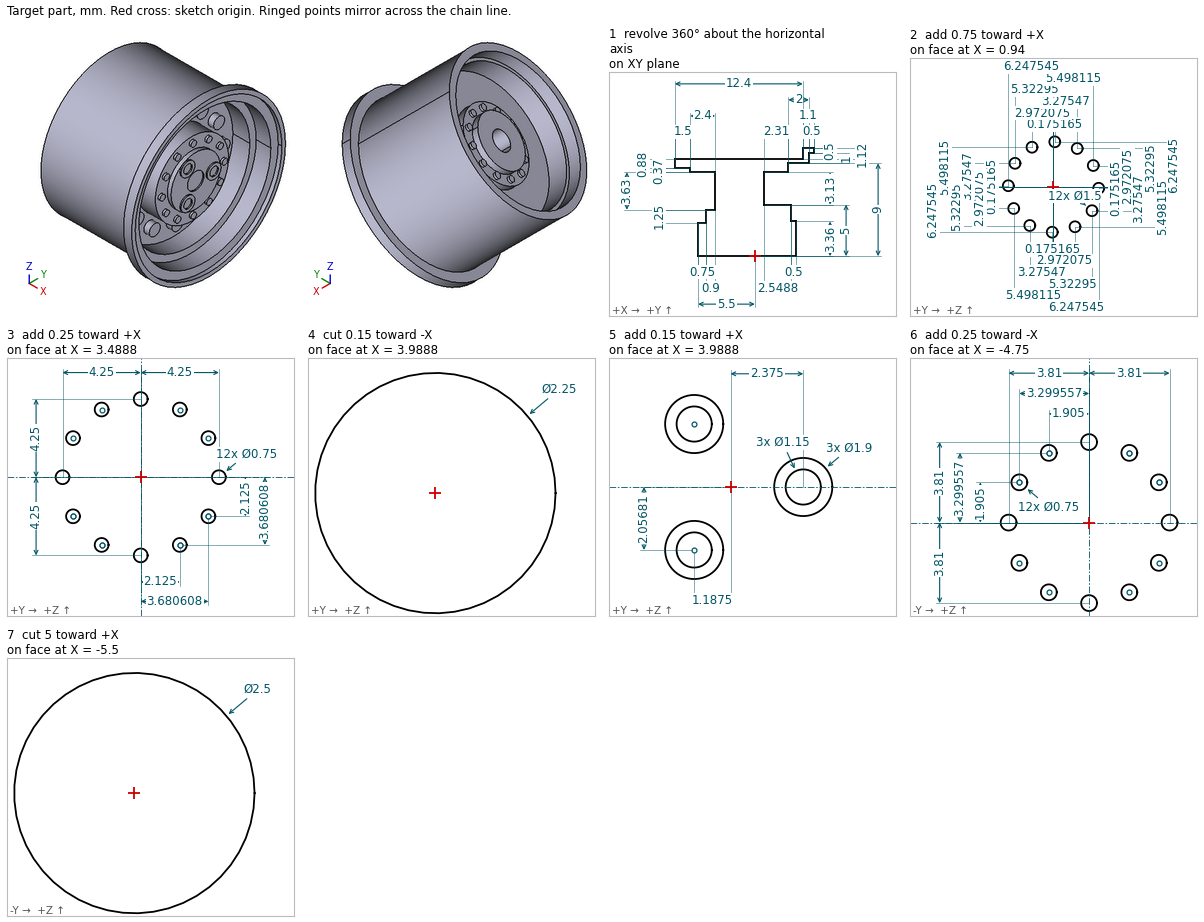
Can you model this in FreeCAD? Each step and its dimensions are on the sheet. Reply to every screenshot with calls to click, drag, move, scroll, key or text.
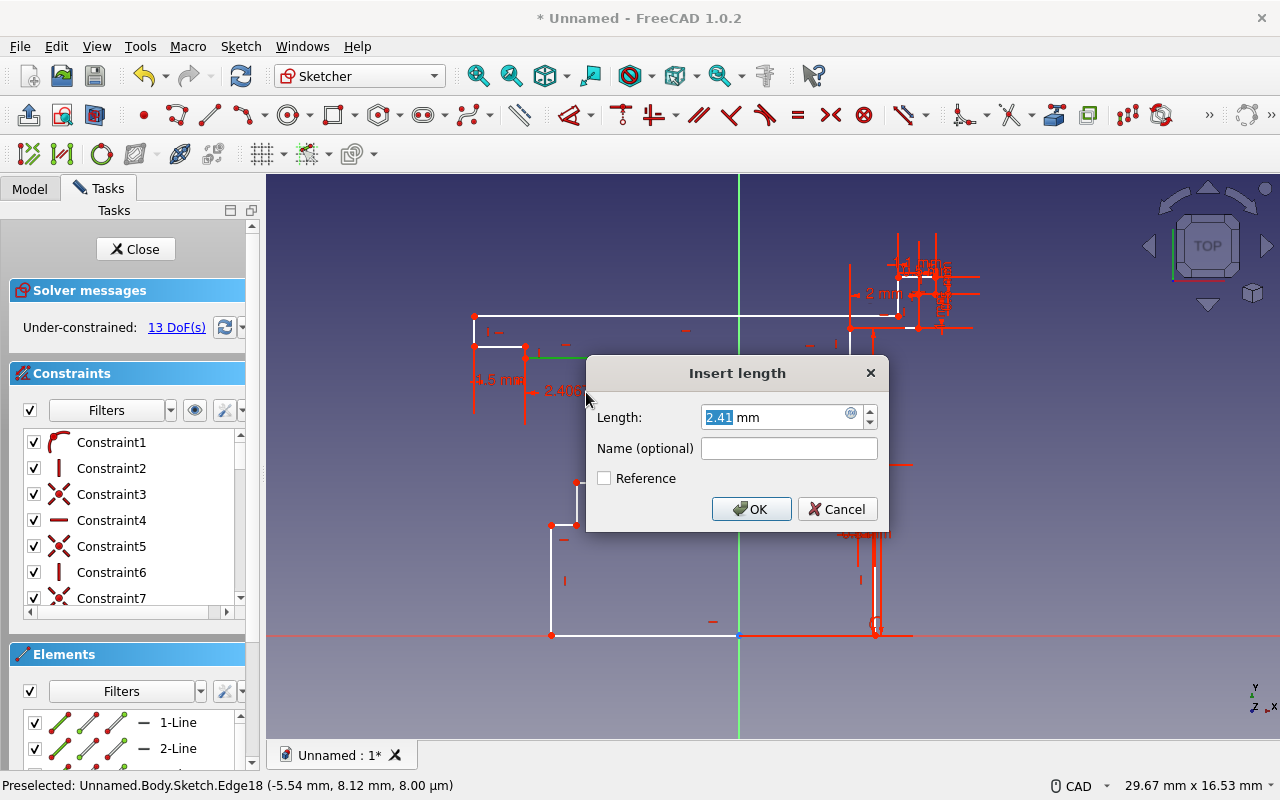
text(2.4)
key(Return)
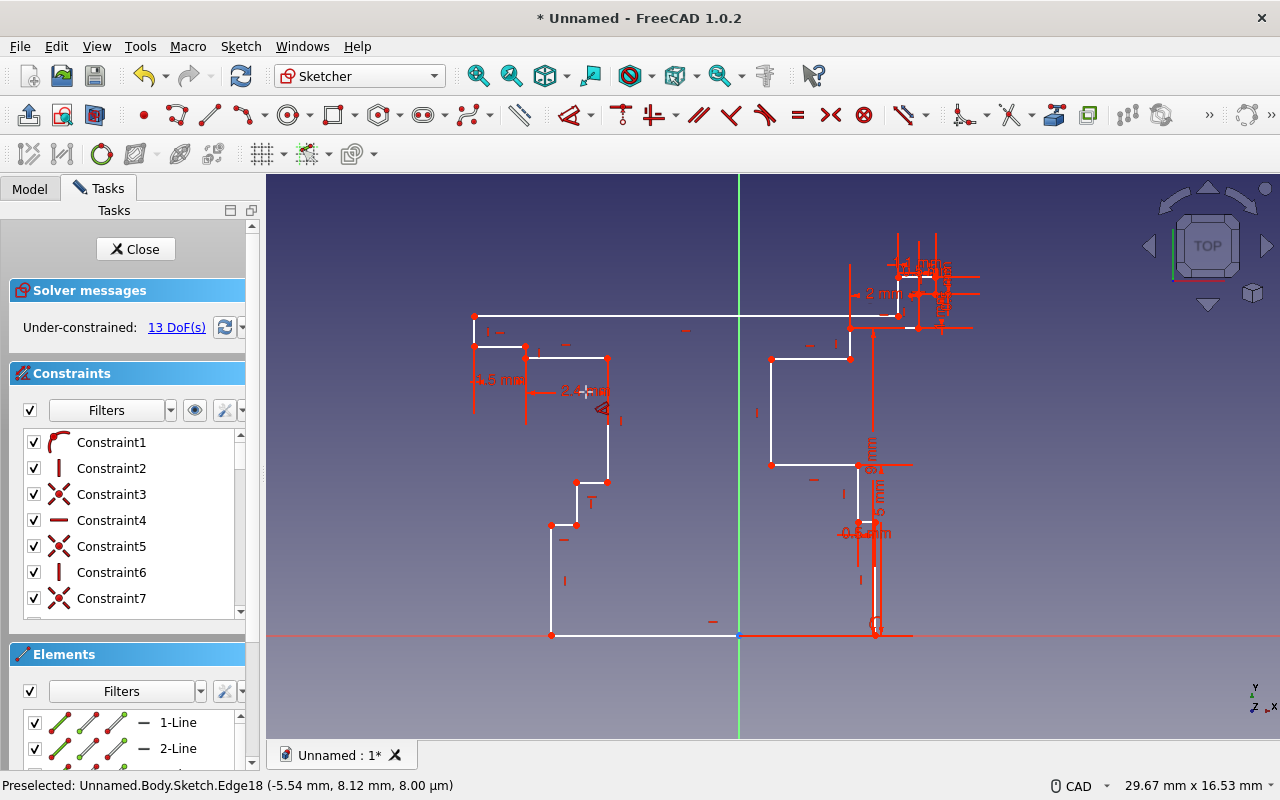
scroll(599, 483, up, 3)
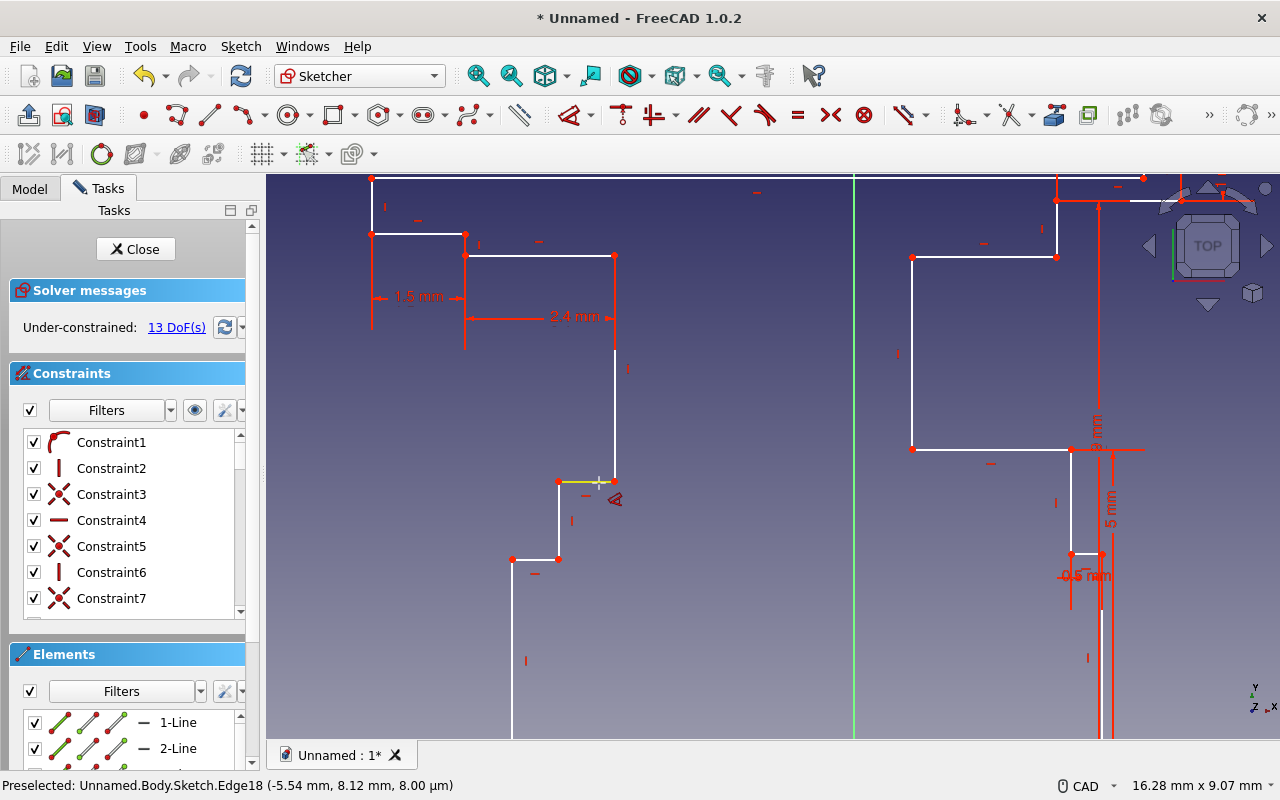
click(598, 482)
click(587, 516)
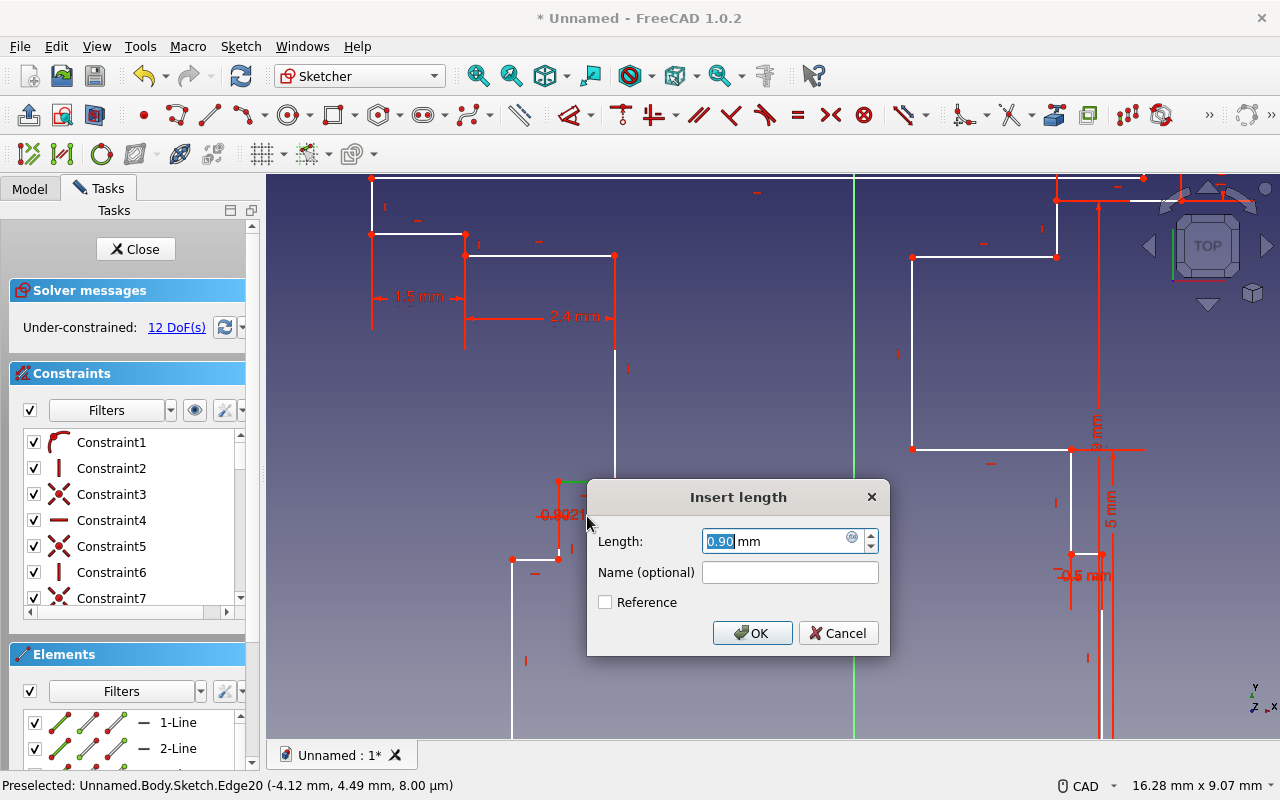
text(0.9)
key(Return)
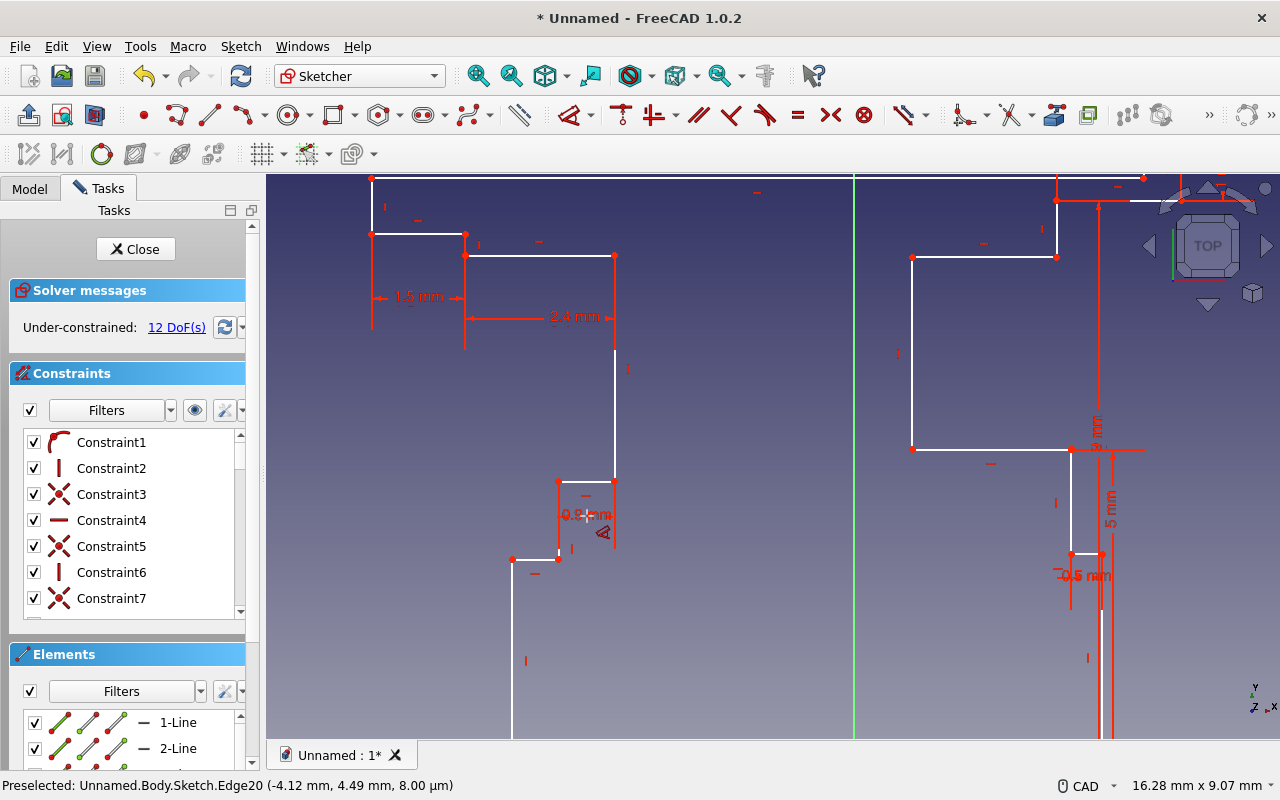
click(1102, 699)
click(1068, 633)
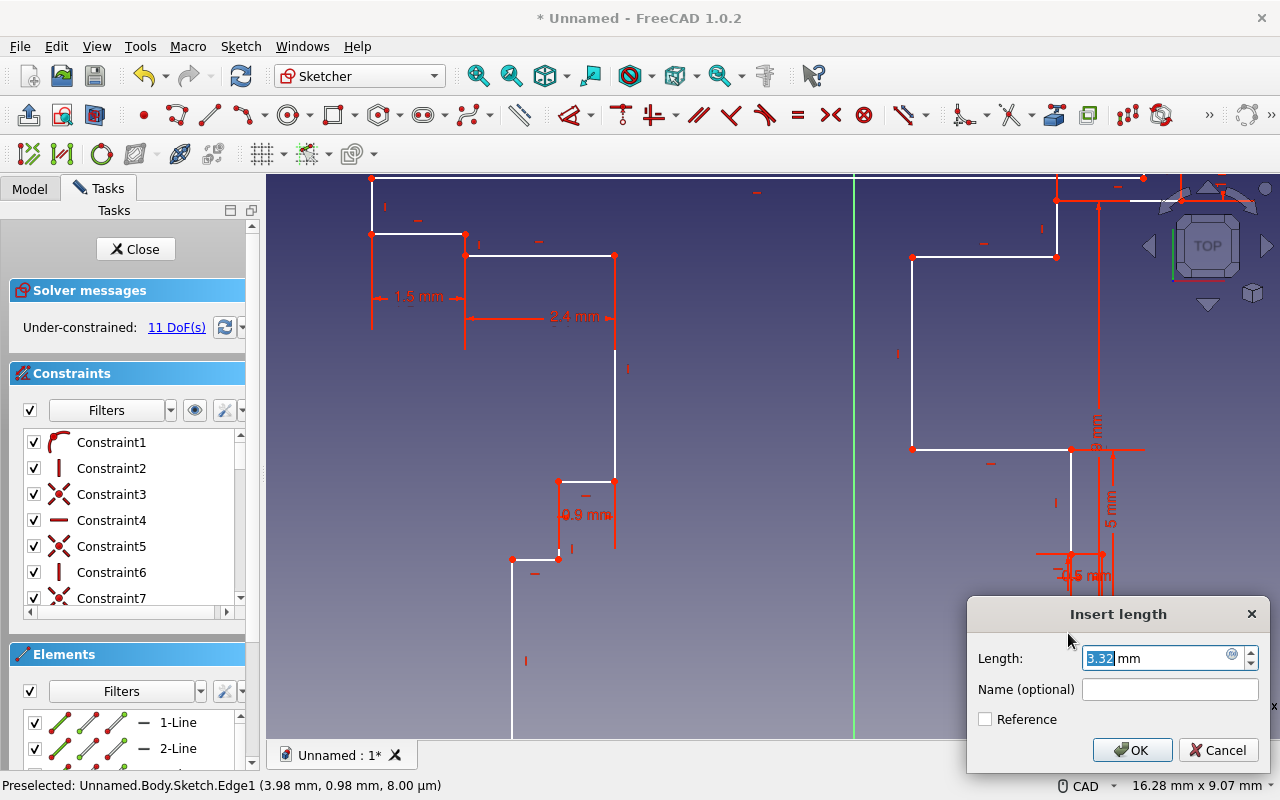
text(3.36)
key(Return)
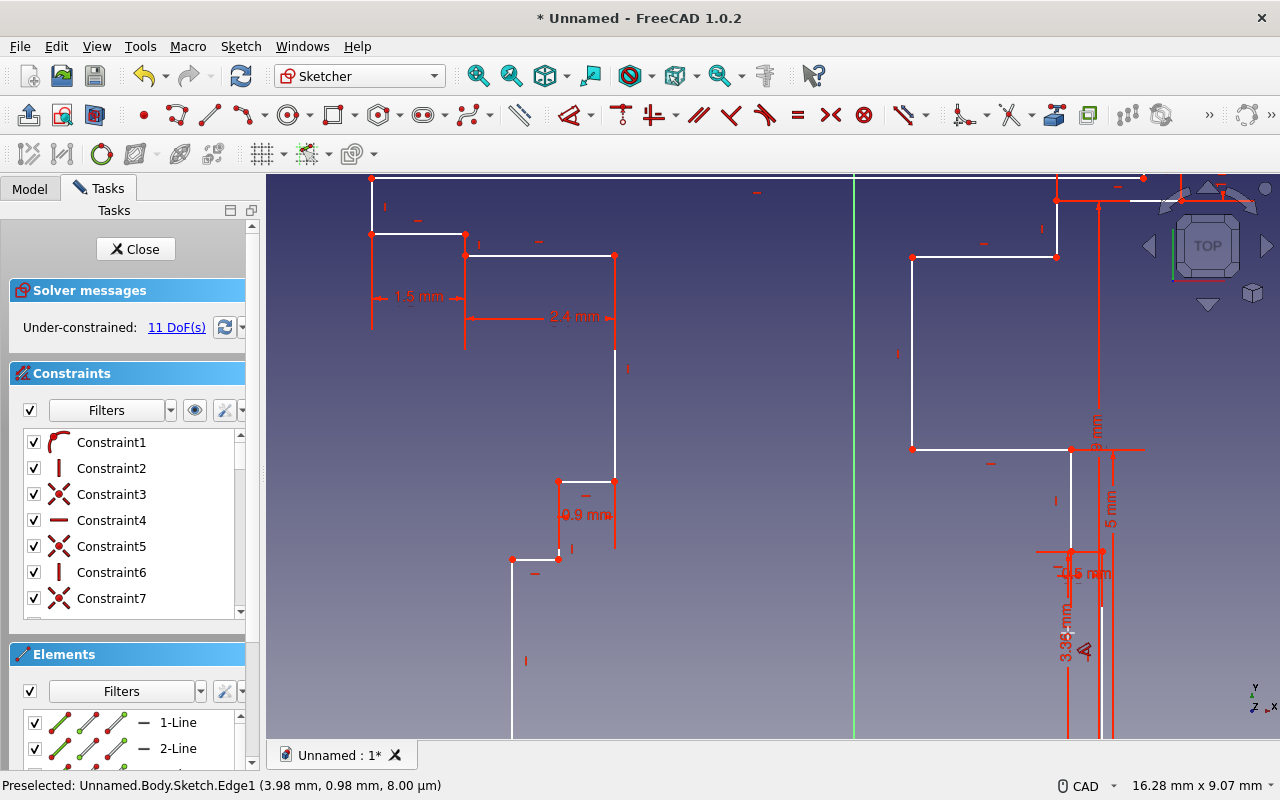
click(912, 392)
click(946, 354)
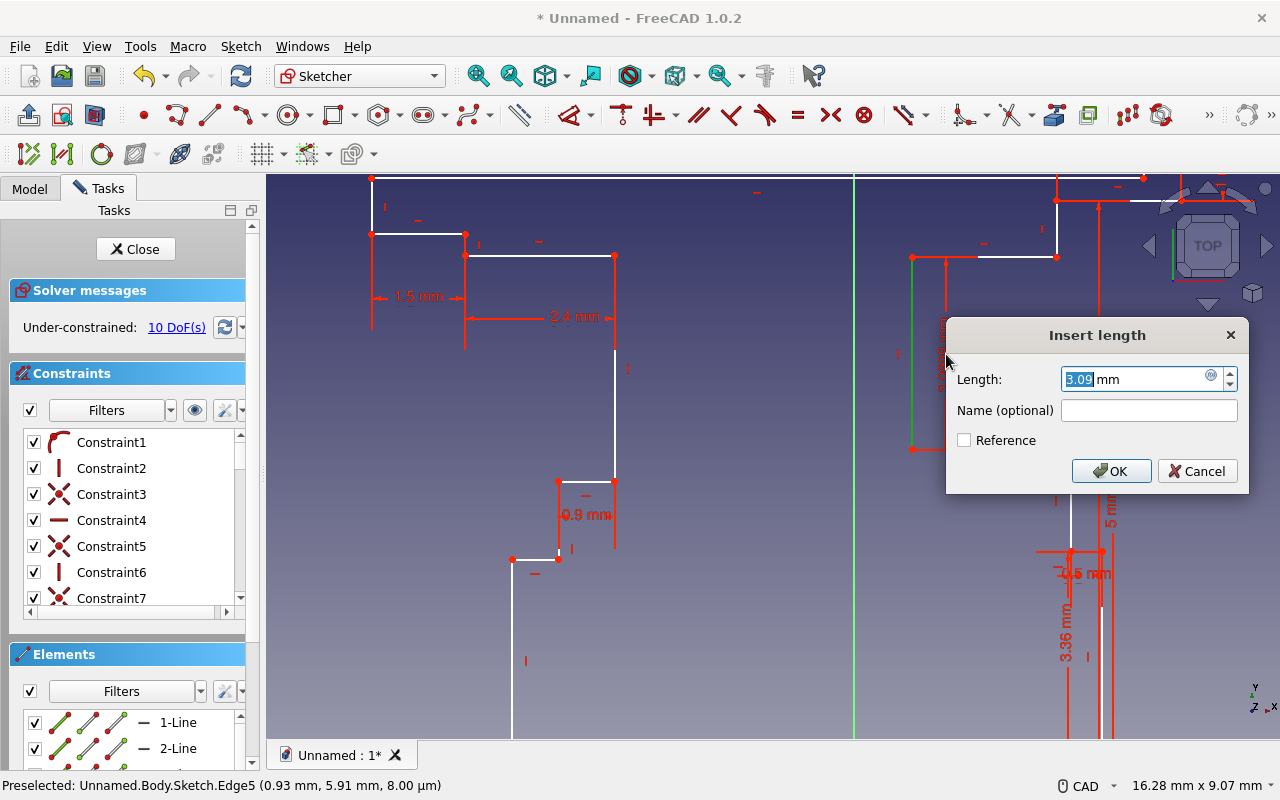
text(3.13)
key(Return)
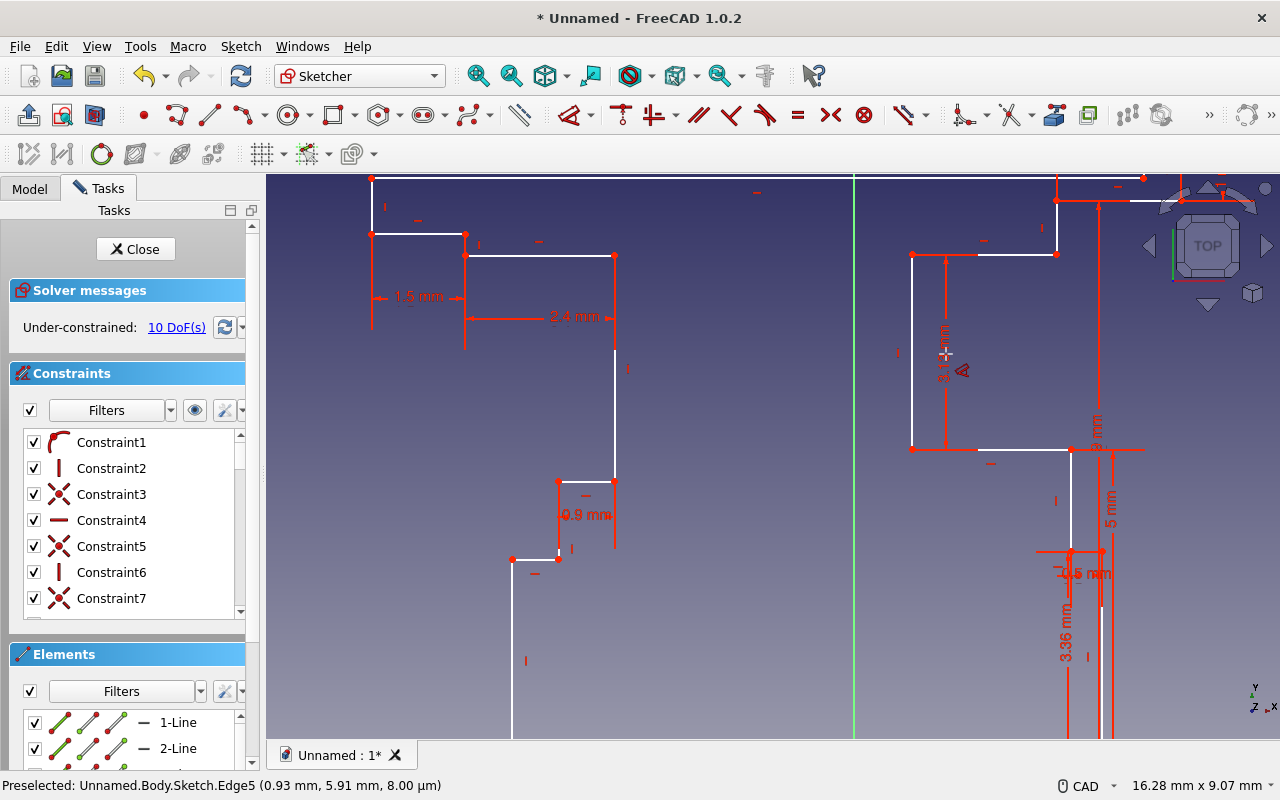
click(956, 255)
click(985, 221)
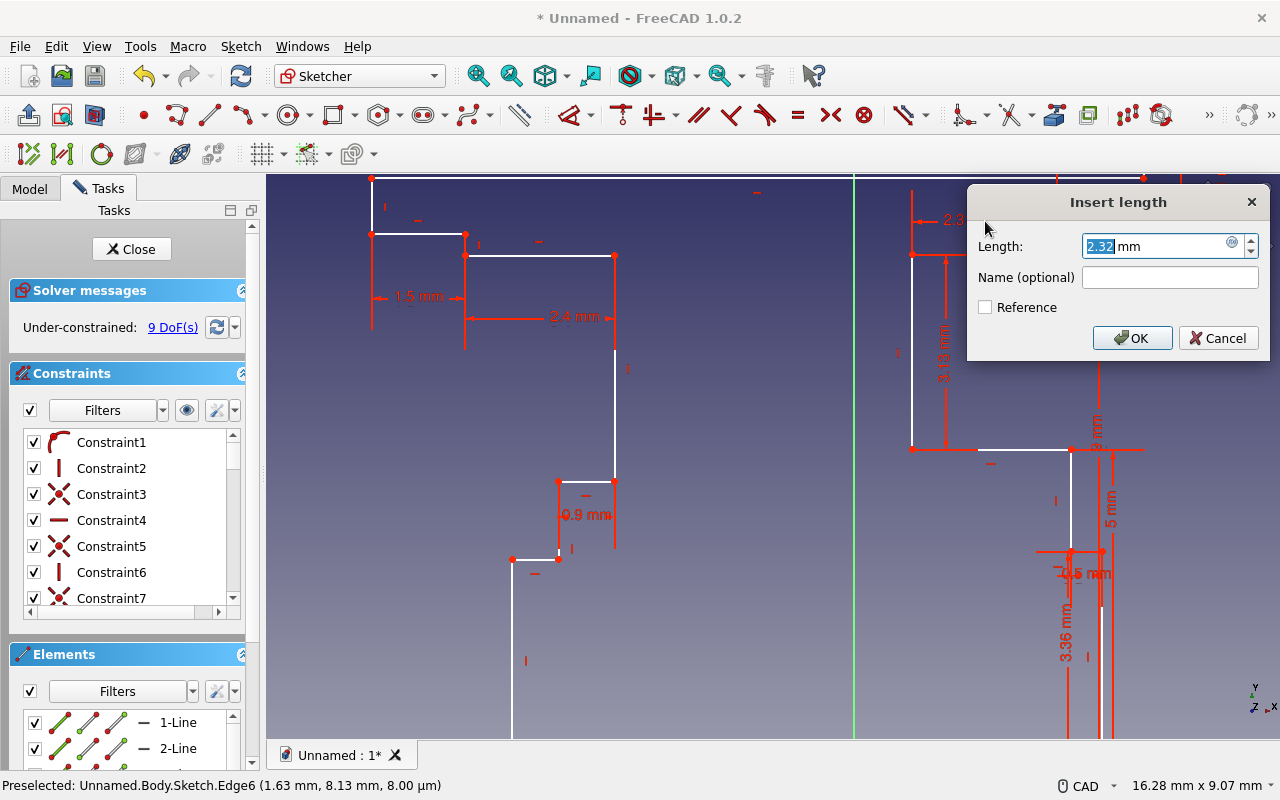
text(2.31)
key(Return)